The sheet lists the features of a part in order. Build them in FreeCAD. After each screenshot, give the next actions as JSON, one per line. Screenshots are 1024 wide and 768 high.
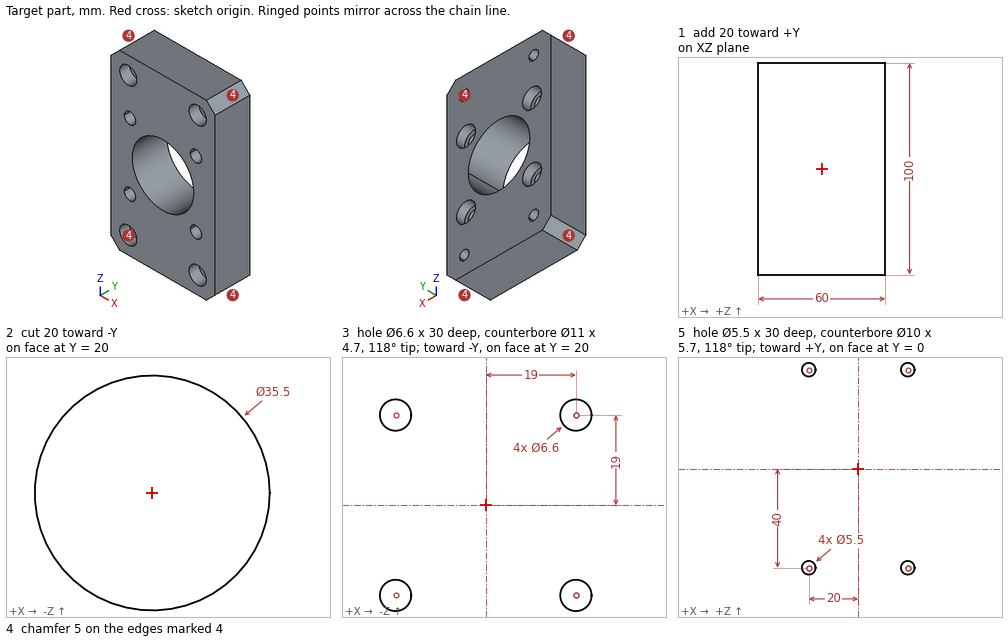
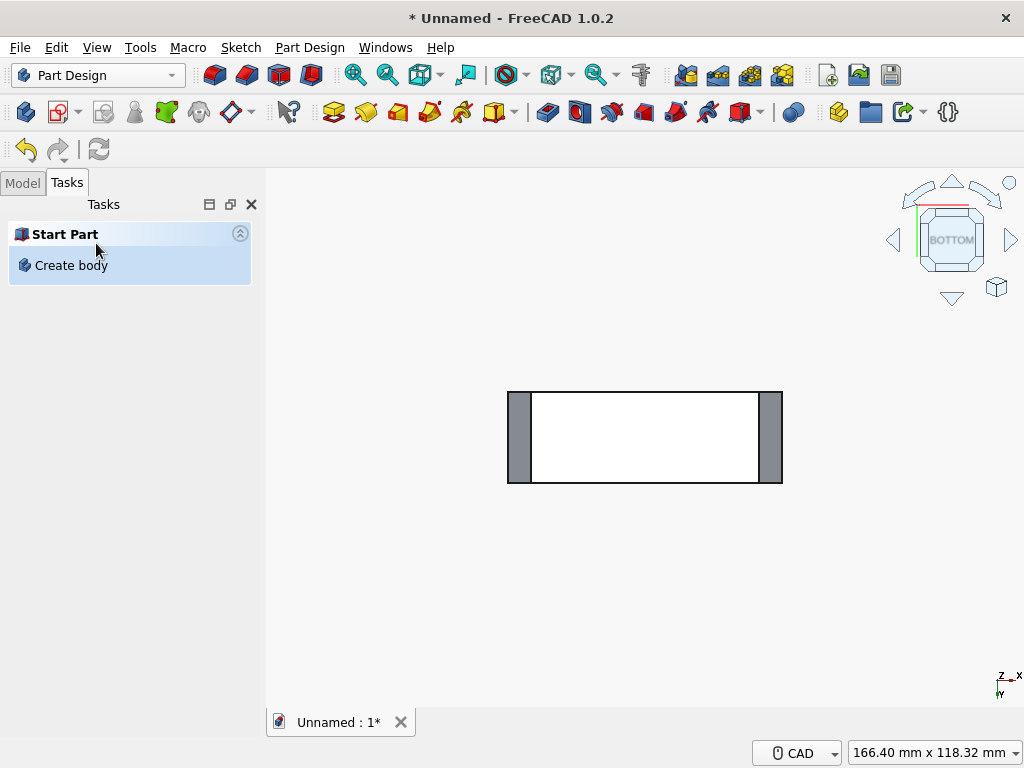
{"action": "left_click", "coordinate": [356, 76]}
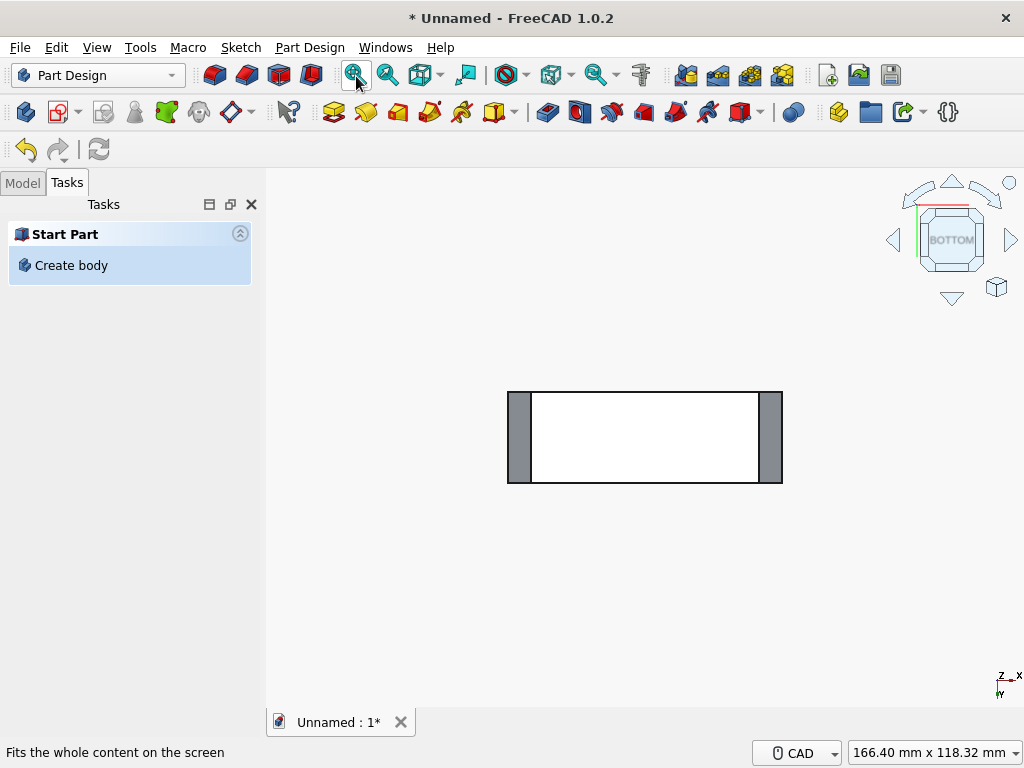
{"action": "key", "text": "0"}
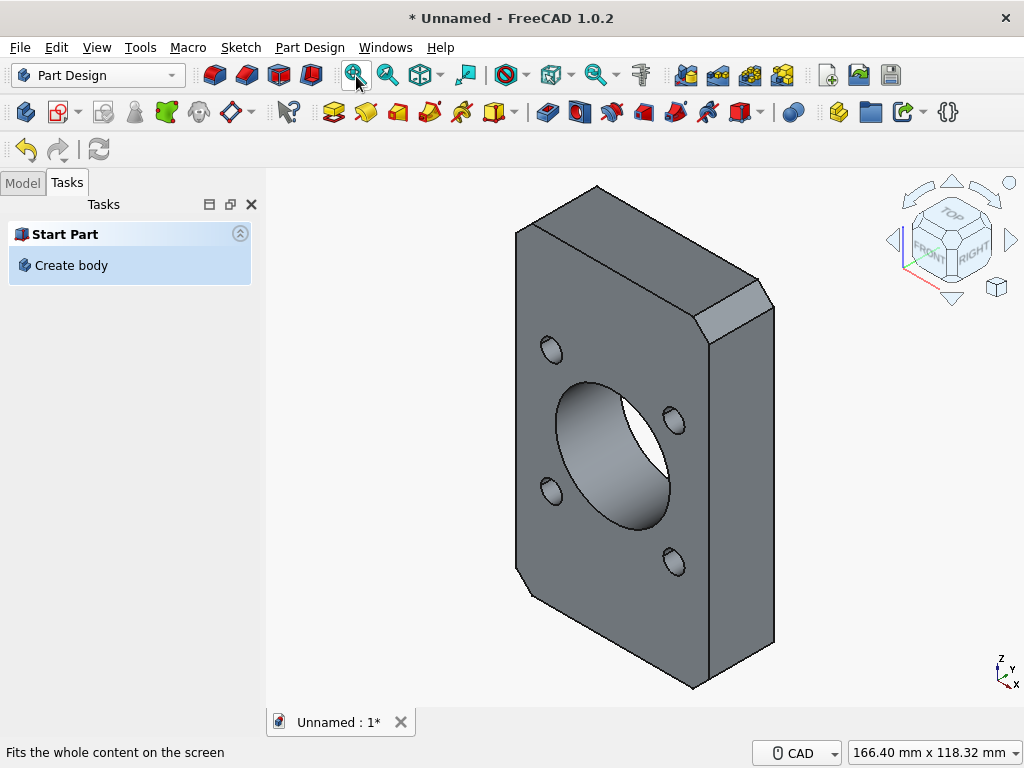
{"action": "left_click", "coordinate": [640, 365]}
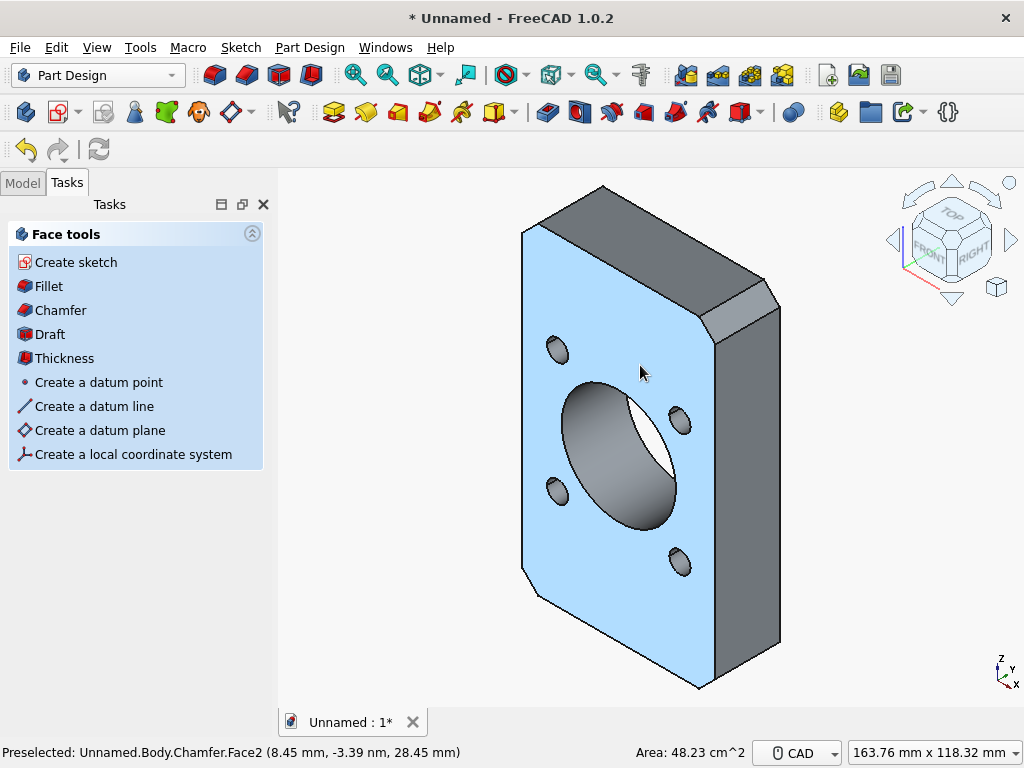
{"action": "left_click", "coordinate": [58, 112]}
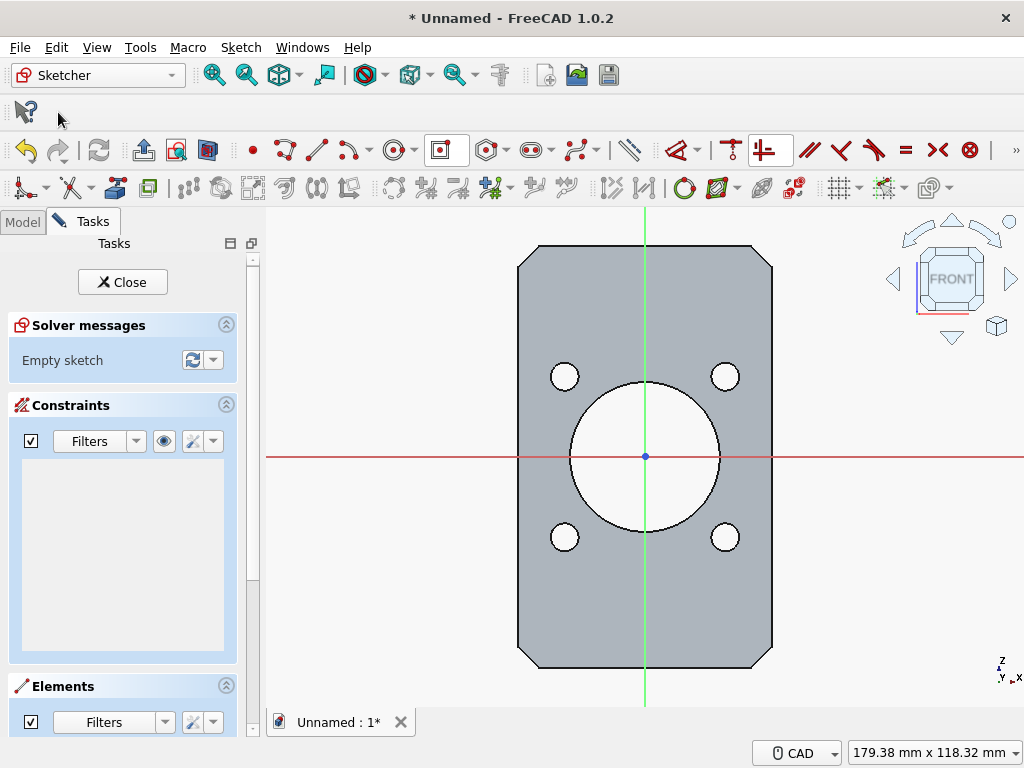
{"action": "left_click", "coordinate": [394, 150]}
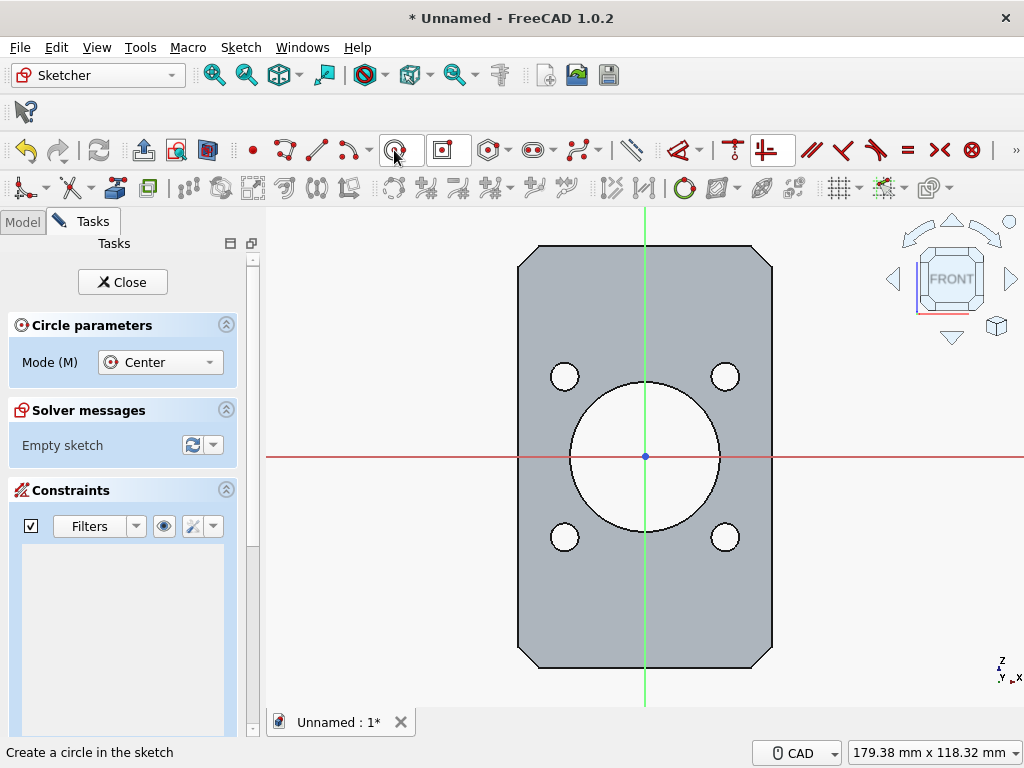
{"action": "scroll", "coordinate": [560, 626], "scroll_direction": "up", "scroll_amount": 4}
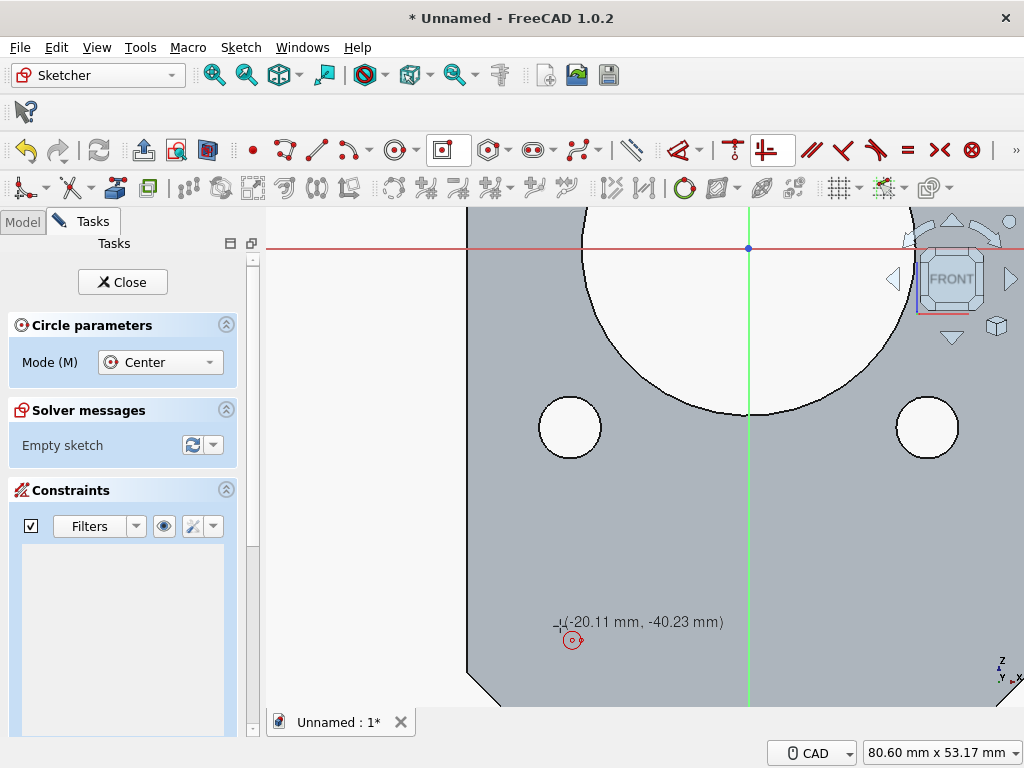
{"action": "left_click", "coordinate": [561, 625]}
{"action": "left_click", "coordinate": [579, 607]}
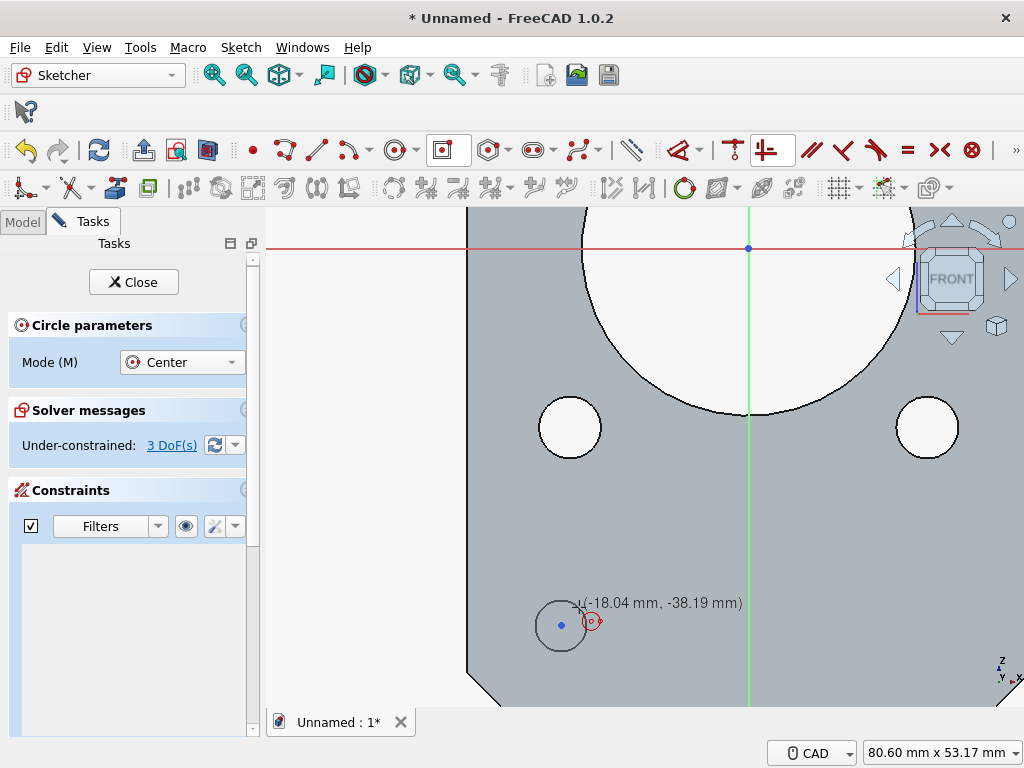
{"action": "scroll", "coordinate": [476, 578], "scroll_direction": "down", "scroll_amount": 5}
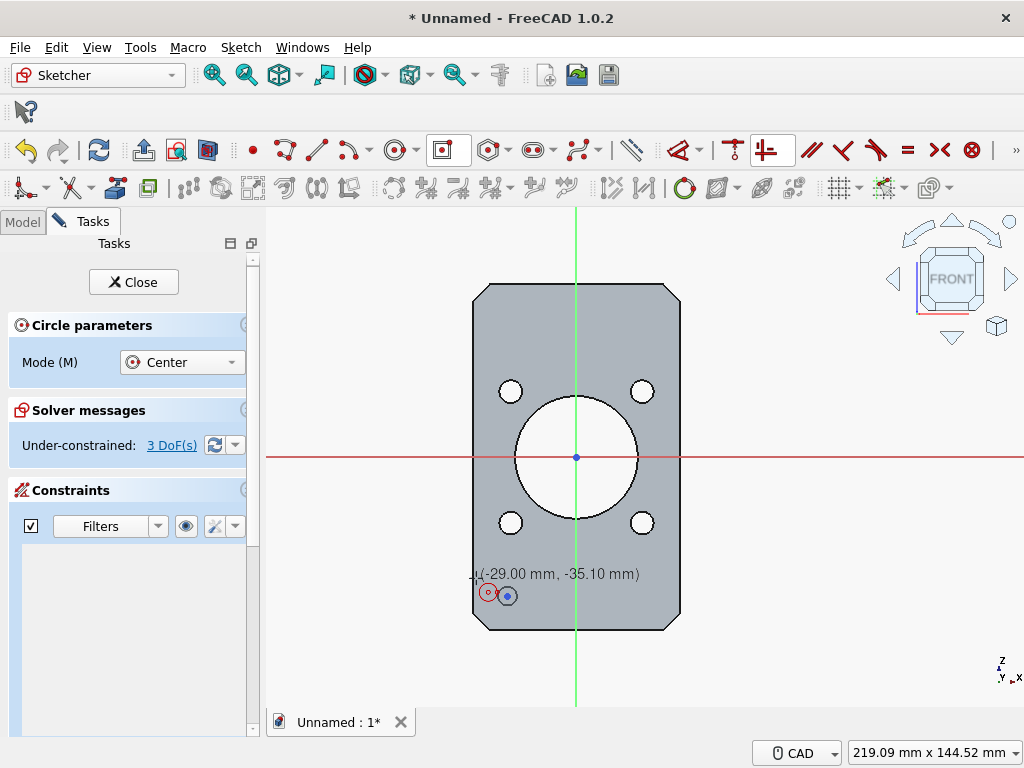
{"action": "scroll", "coordinate": [646, 596], "scroll_direction": "up", "scroll_amount": 5}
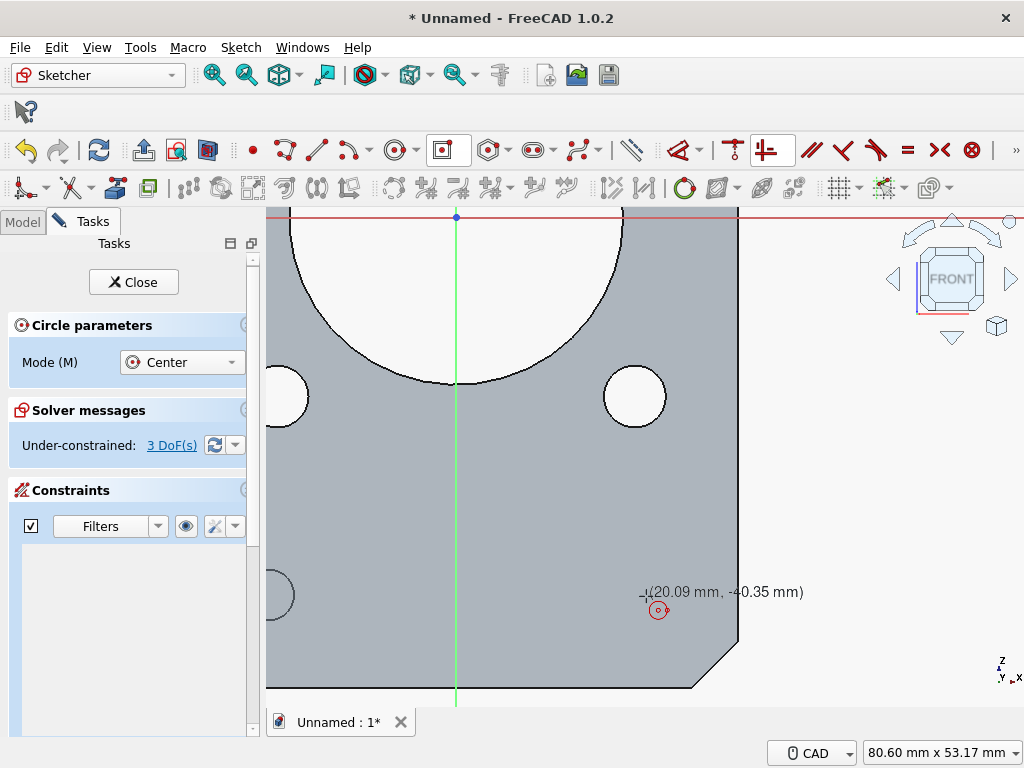
{"action": "left_click", "coordinate": [644, 594]}
{"action": "left_click", "coordinate": [663, 576]}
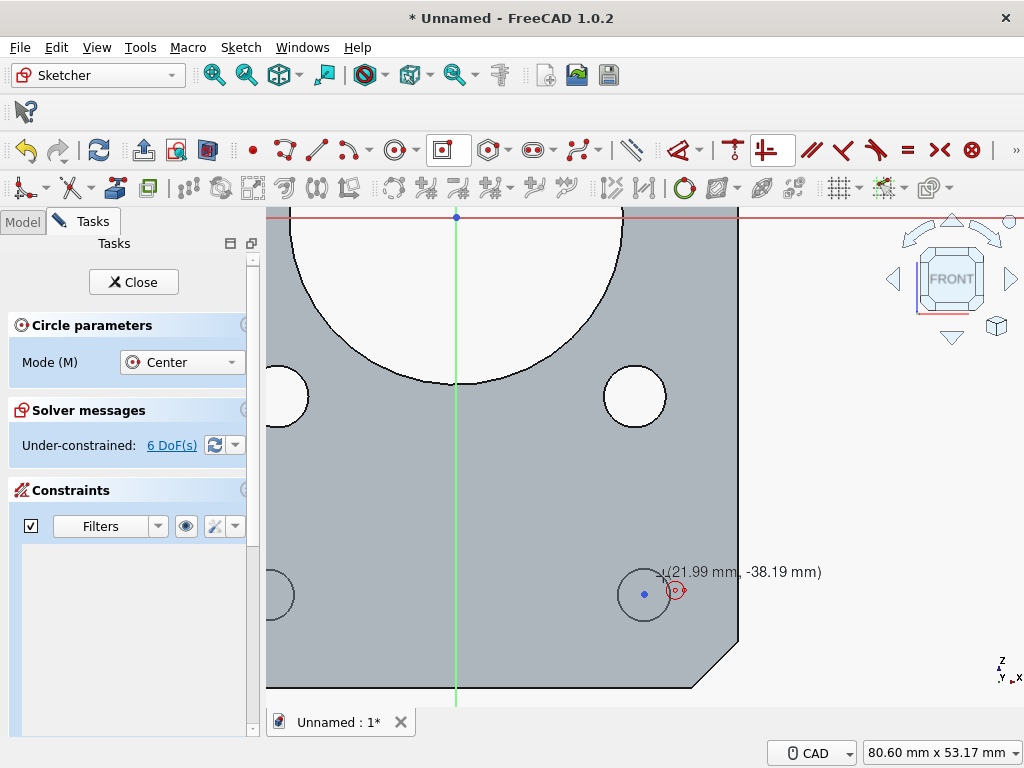
{"action": "scroll", "coordinate": [647, 596], "scroll_direction": "down", "scroll_amount": 5}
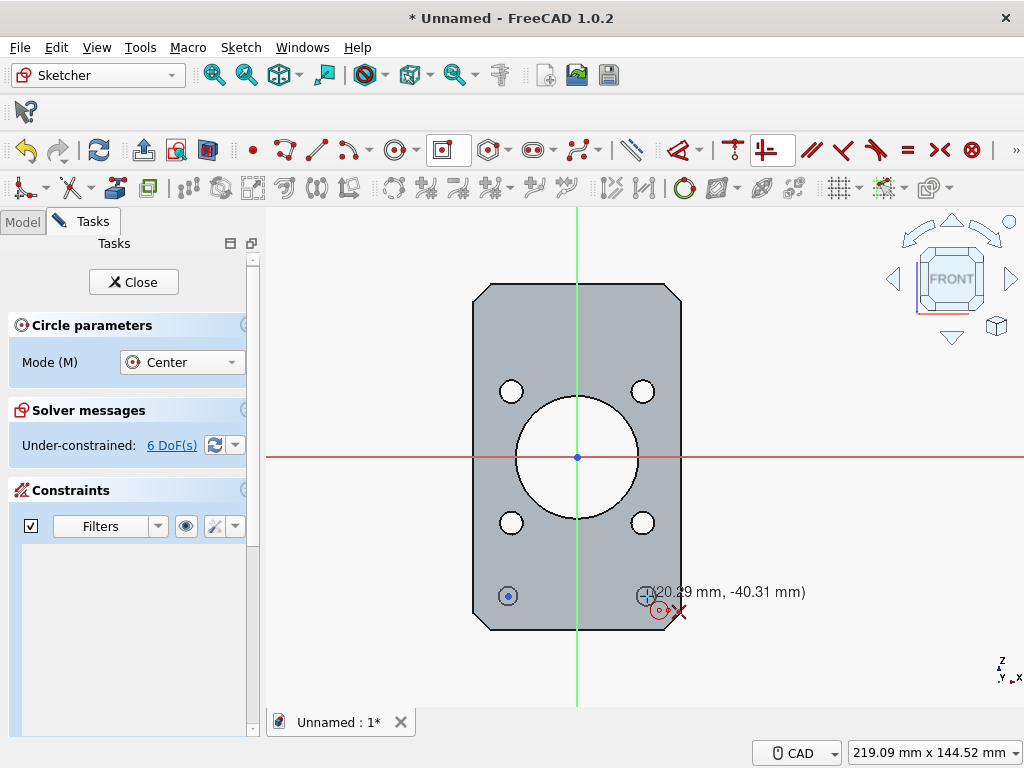
{"action": "scroll", "coordinate": [508, 319], "scroll_direction": "up", "scroll_amount": 5}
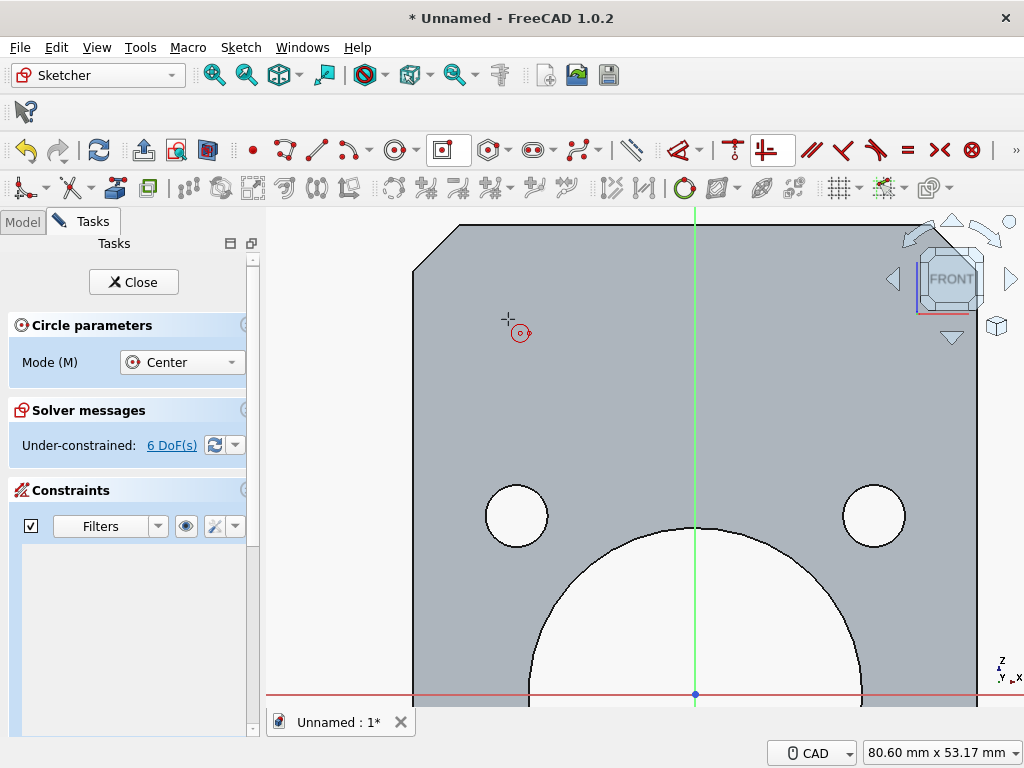
{"action": "left_click", "coordinate": [507, 319]}
{"action": "left_click", "coordinate": [526, 300]}